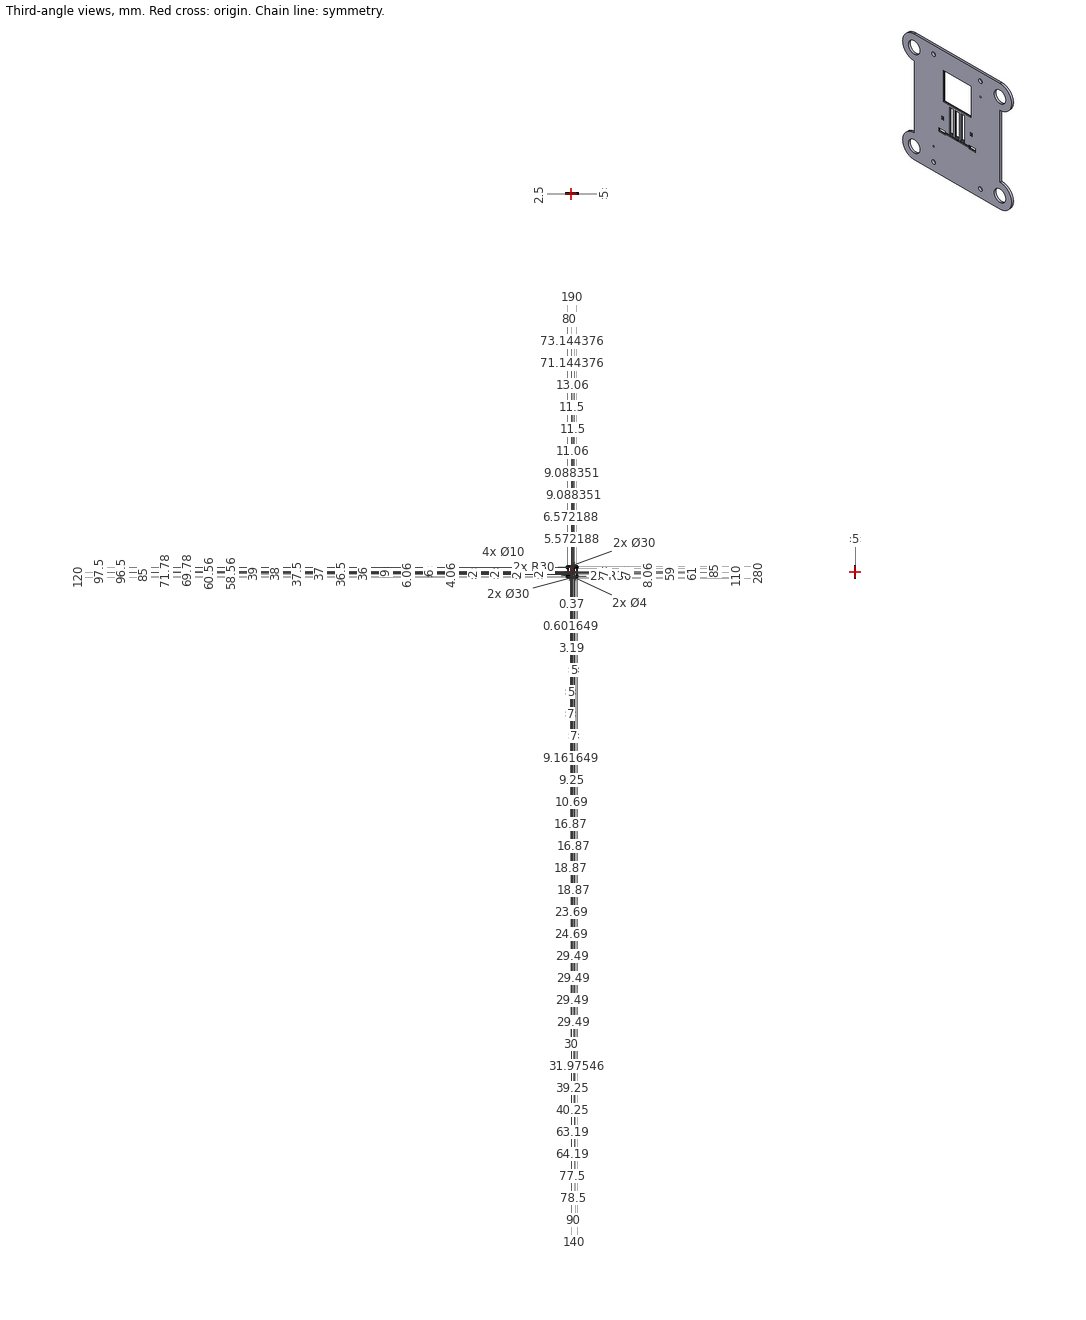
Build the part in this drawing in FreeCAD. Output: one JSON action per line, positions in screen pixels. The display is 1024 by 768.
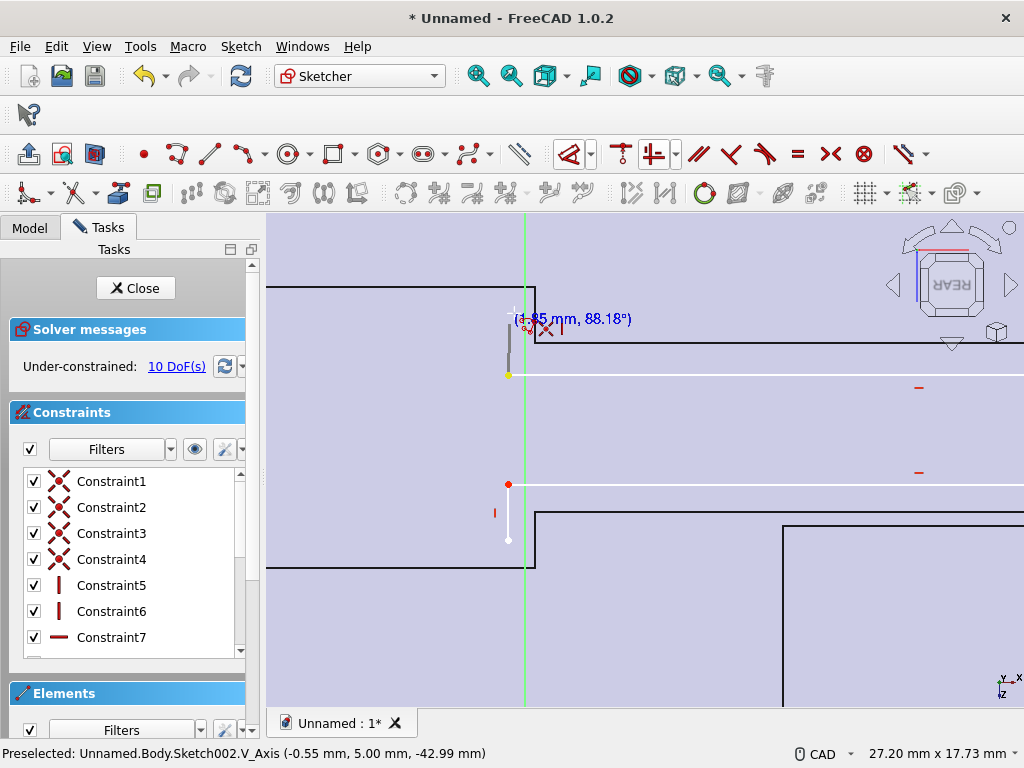
{"action": "left_click", "coordinate": [508, 315]}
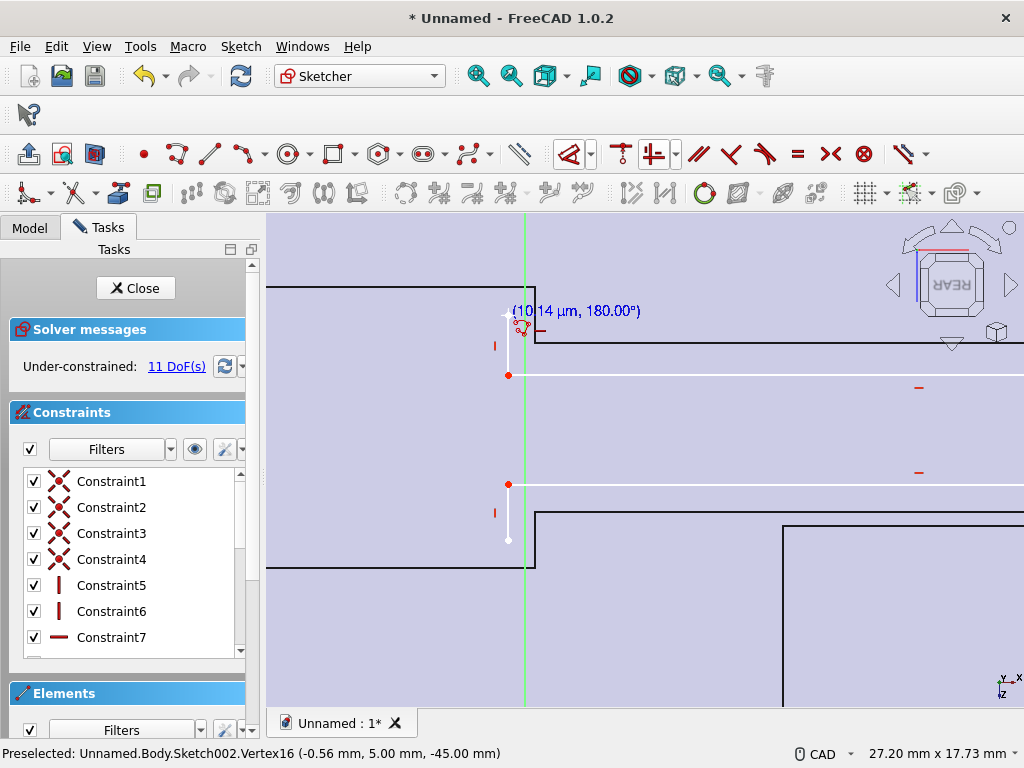
{"action": "scroll", "coordinate": [514, 313], "scroll_direction": "down", "scroll_amount": 13}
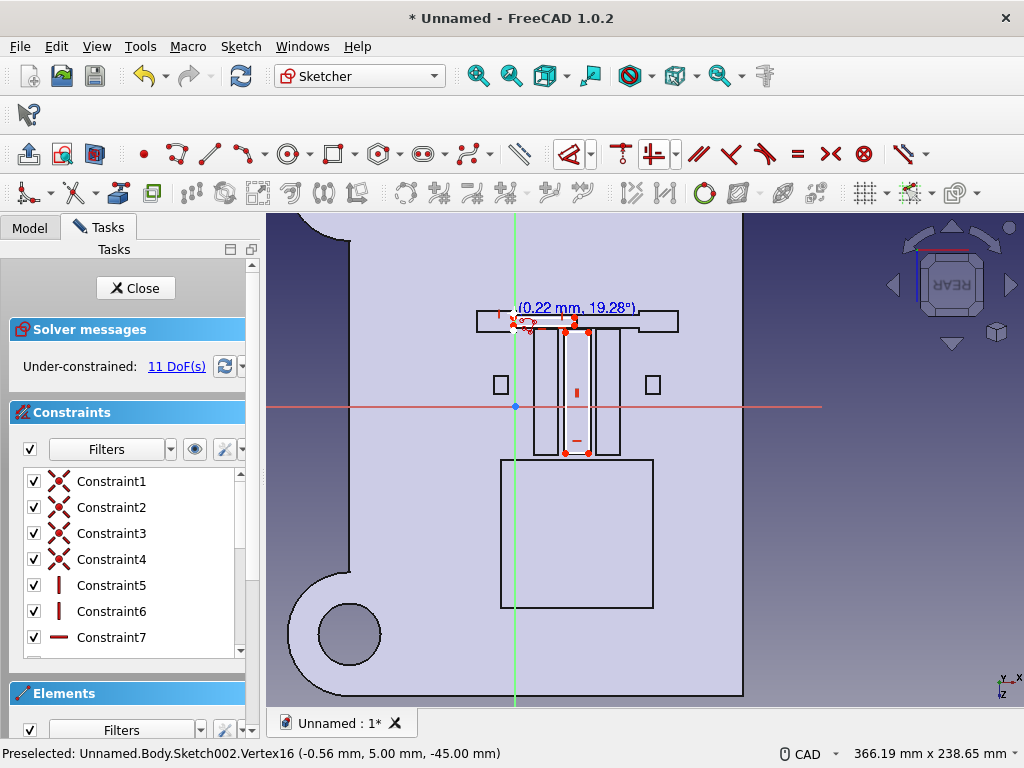
{"action": "left_click", "coordinate": [479, 313]}
{"action": "left_click", "coordinate": [479, 330]}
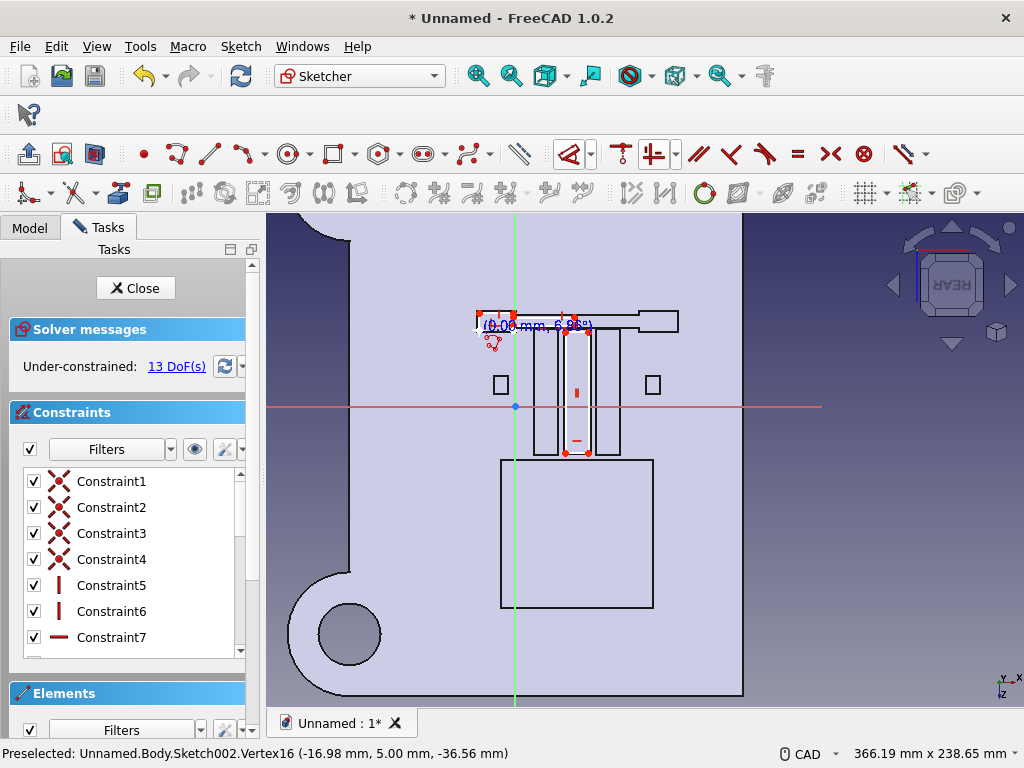
{"action": "scroll", "coordinate": [514, 330], "scroll_direction": "up", "scroll_amount": 13}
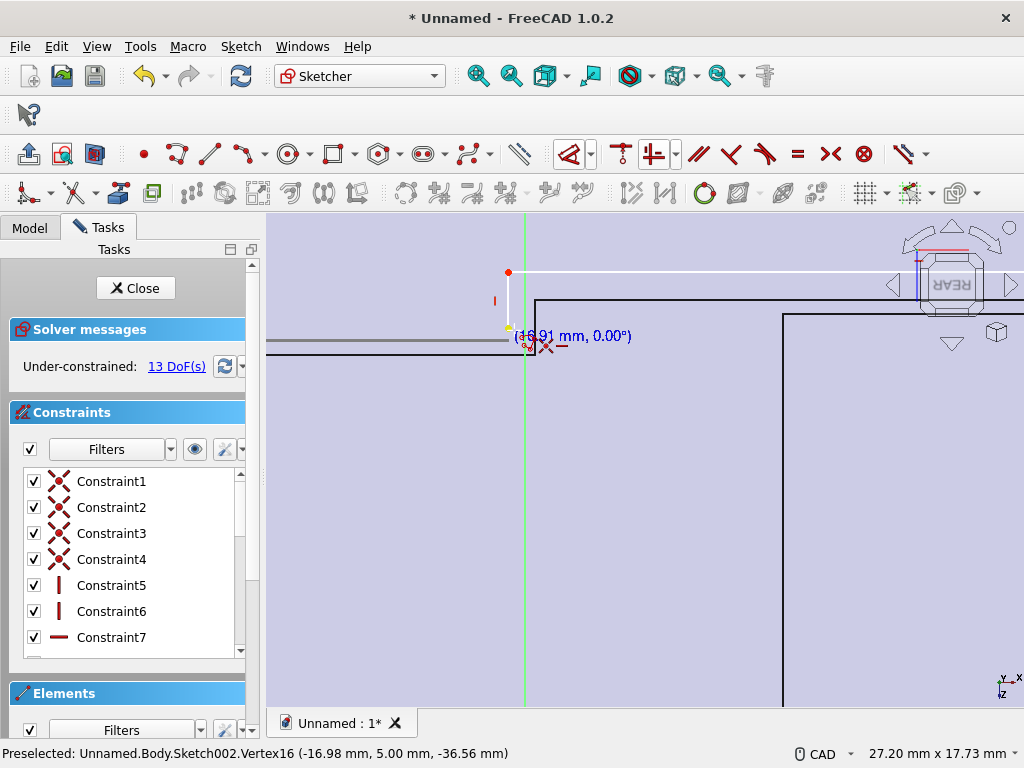
{"action": "left_click", "coordinate": [508, 328]}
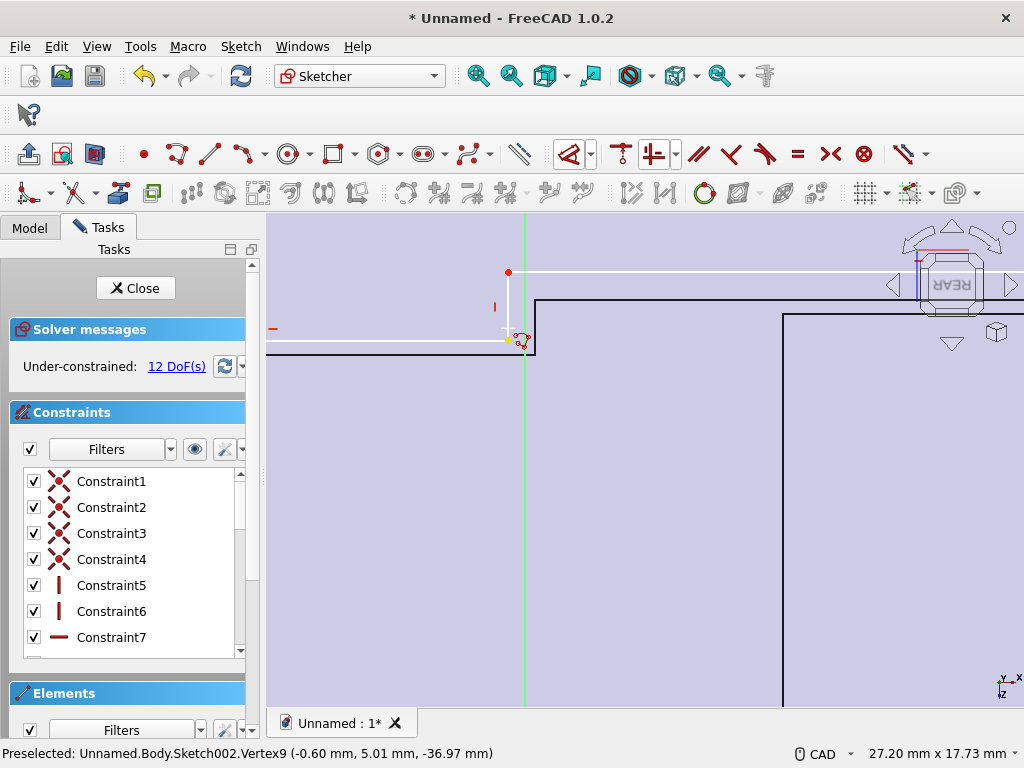
{"action": "scroll", "coordinate": [514, 330], "scroll_direction": "down", "scroll_amount": 13}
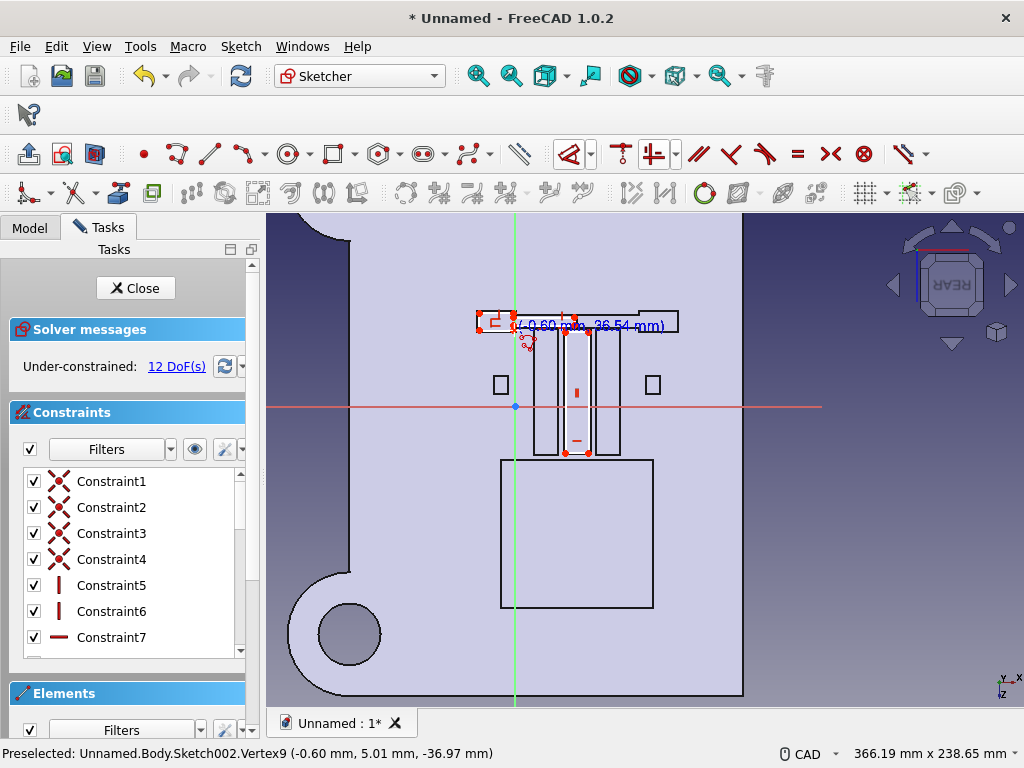
{"action": "scroll", "coordinate": [580, 326], "scroll_direction": "up", "scroll_amount": 7}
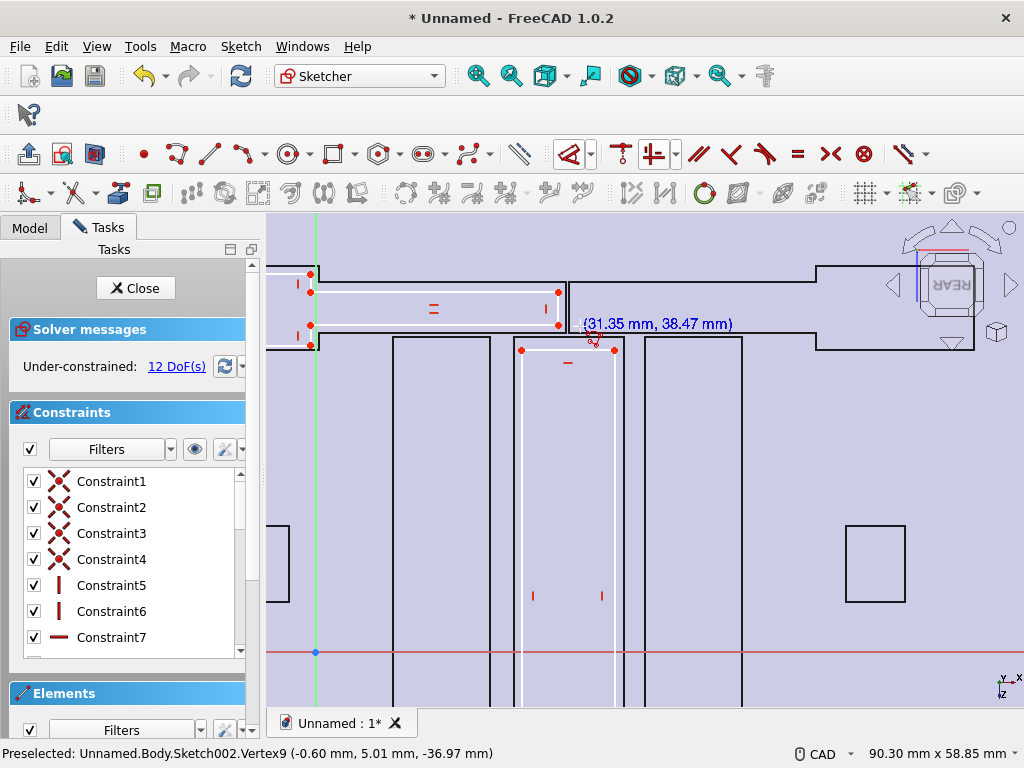
{"action": "left_click", "coordinate": [577, 325]}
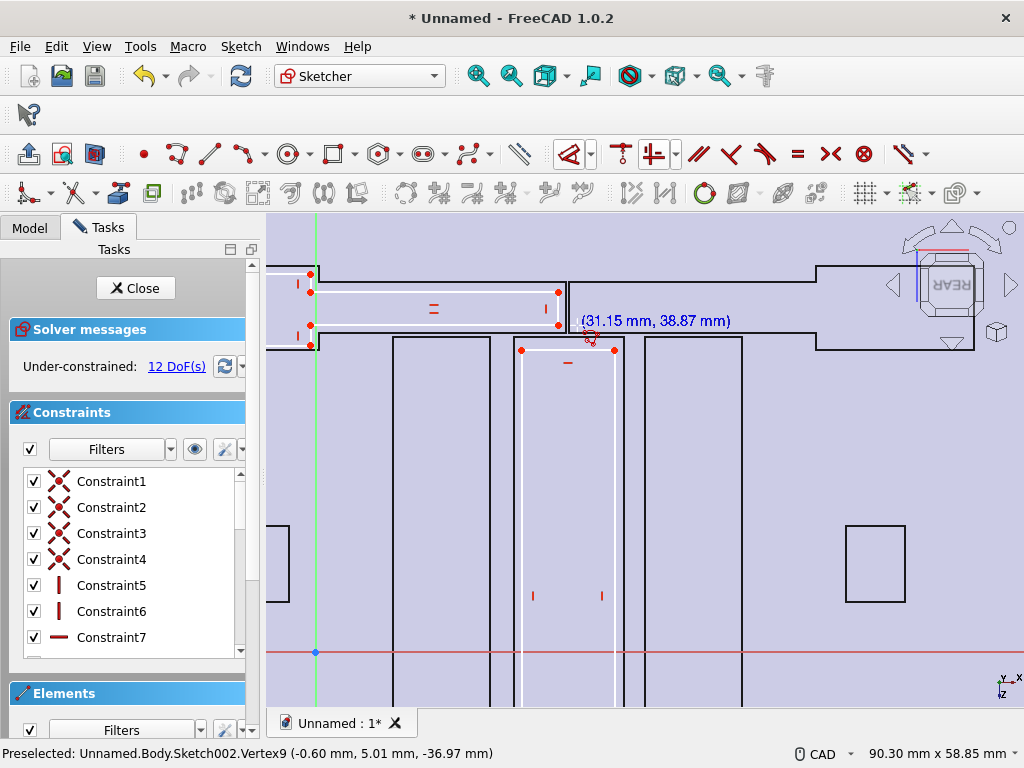
{"action": "scroll", "coordinate": [579, 326], "scroll_direction": "down", "scroll_amount": 7}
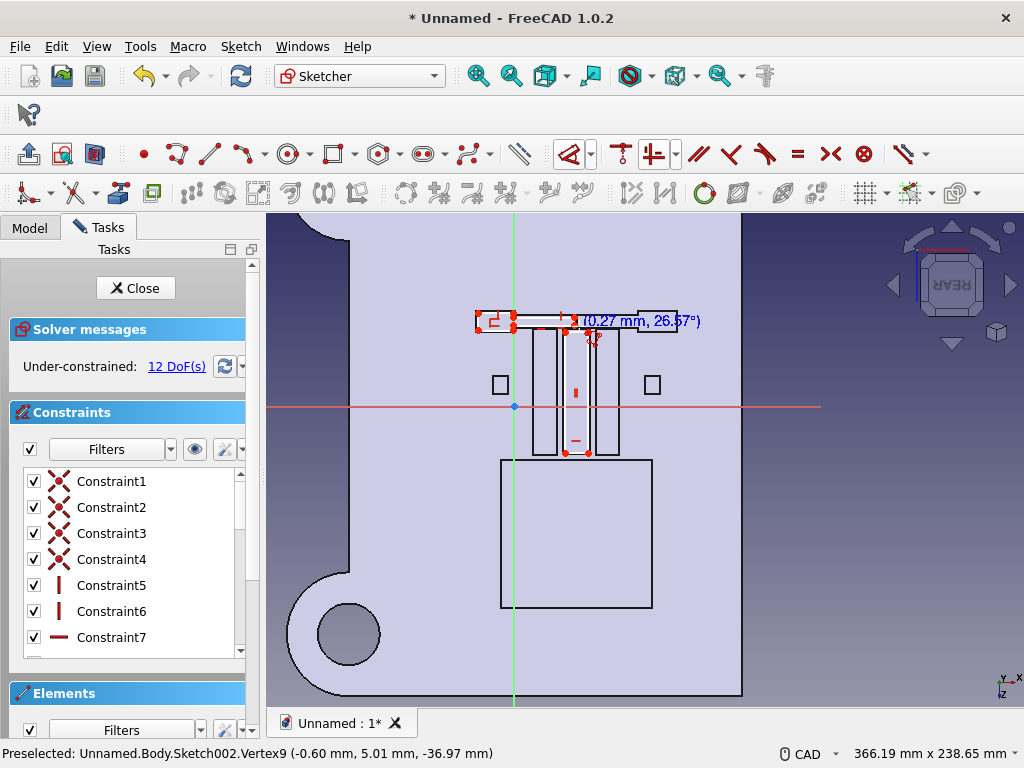
{"action": "left_click", "coordinate": [640, 326]}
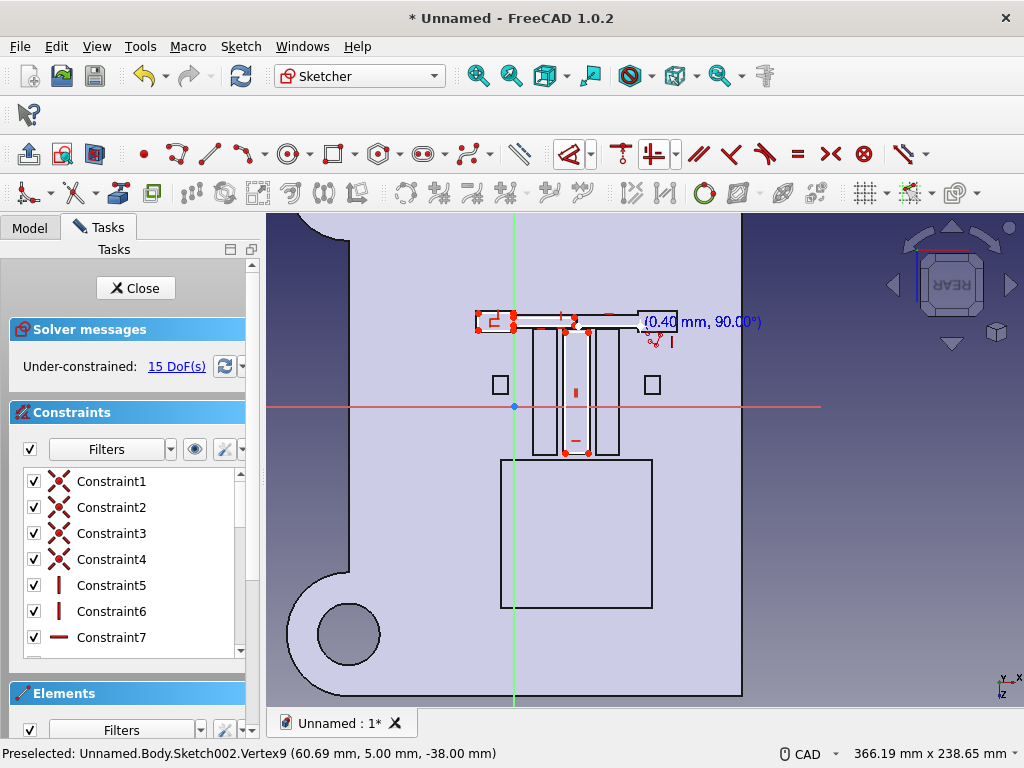
{"action": "scroll", "coordinate": [640, 330], "scroll_direction": "up", "scroll_amount": 7}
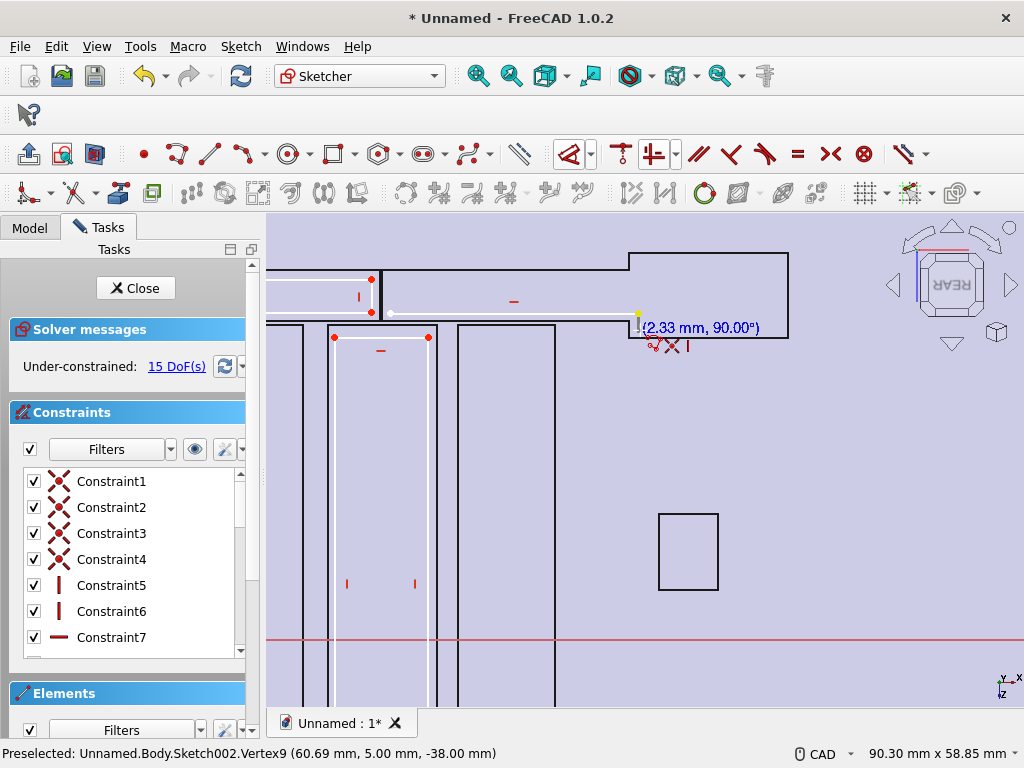
{"action": "left_click", "coordinate": [638, 329]}